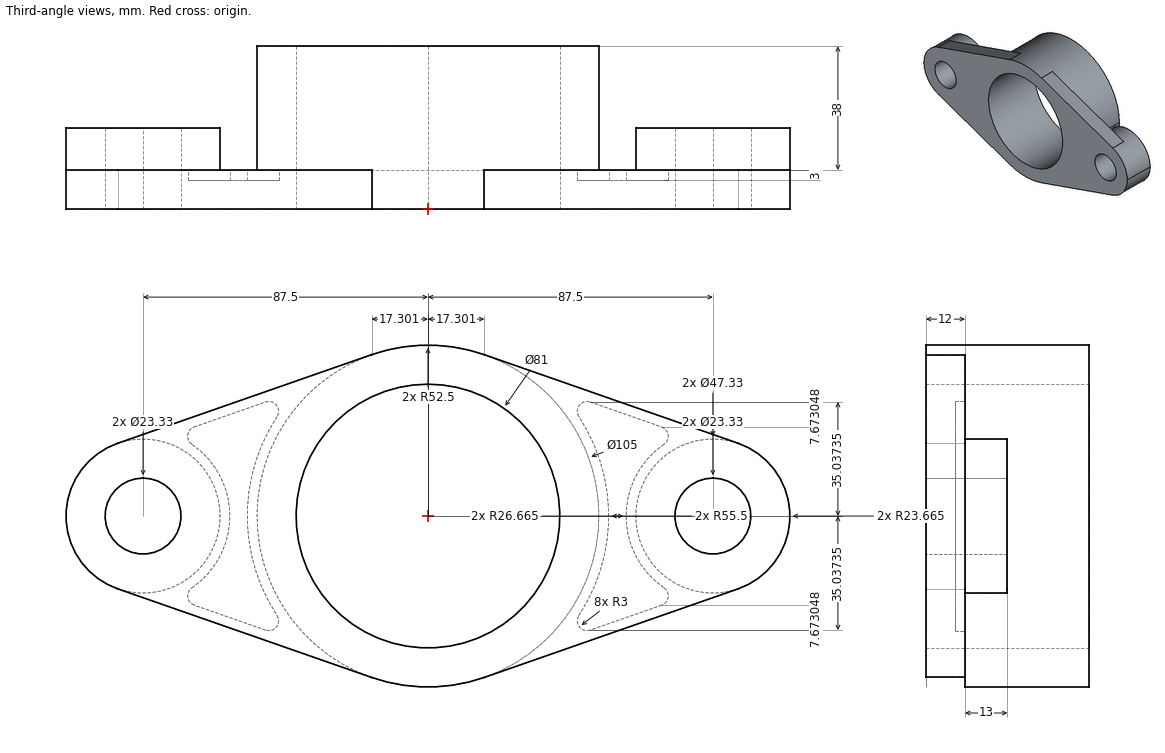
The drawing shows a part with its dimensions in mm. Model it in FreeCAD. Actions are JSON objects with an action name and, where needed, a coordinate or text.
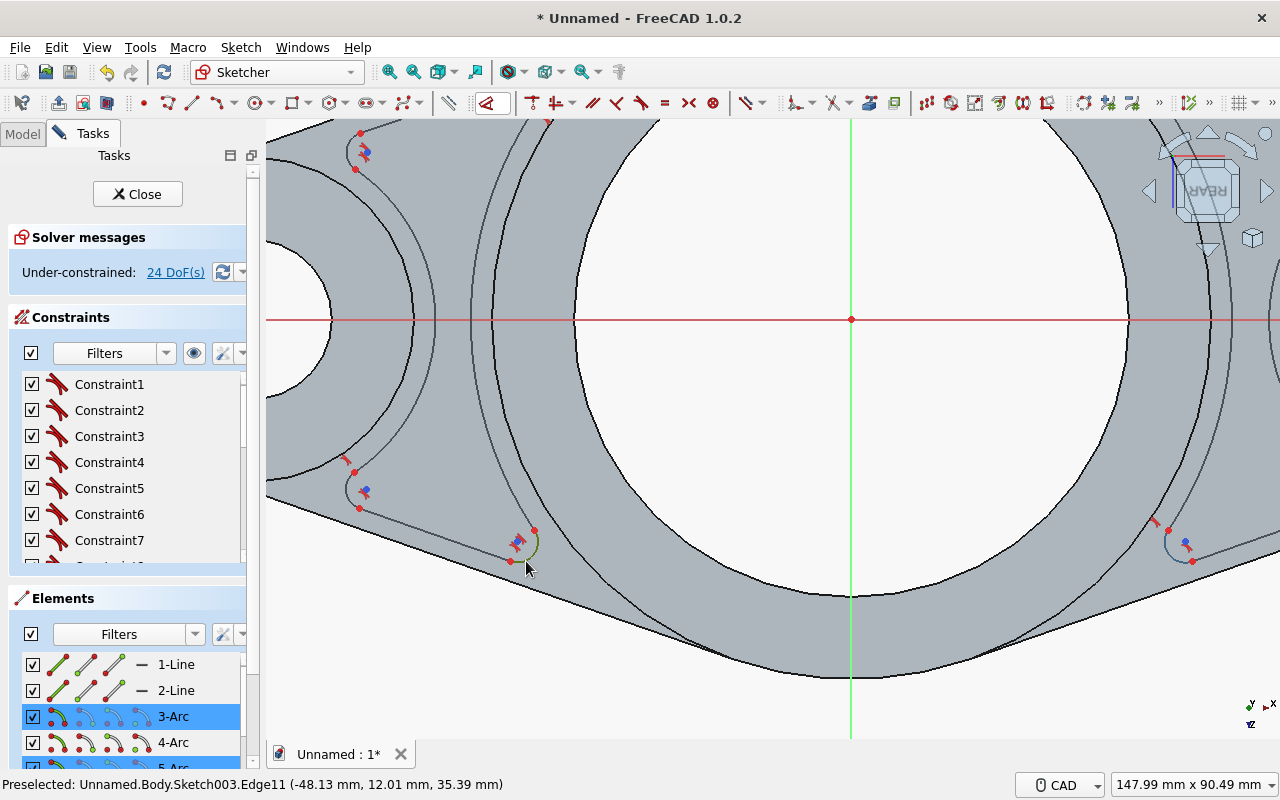
{"action": "scroll", "coordinate": [526, 562], "scroll_direction": "down", "scroll_amount": 3}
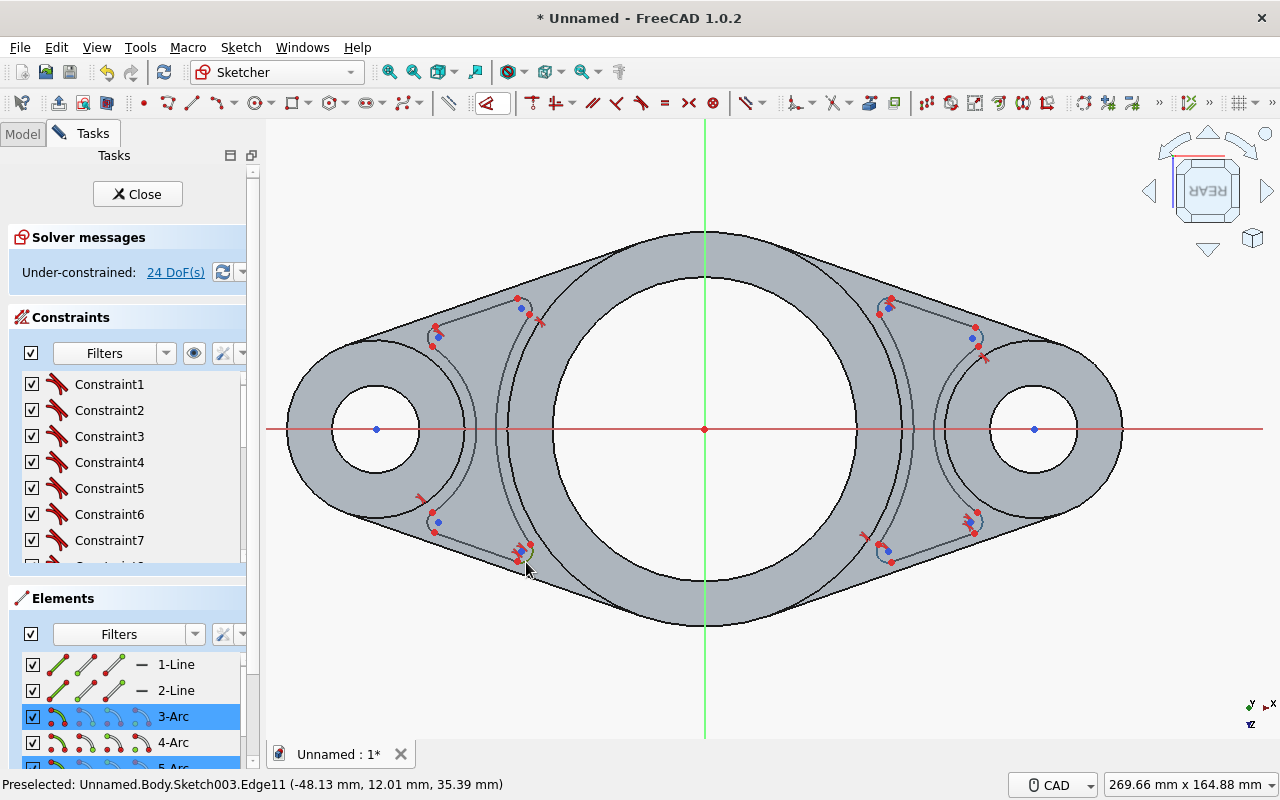
{"action": "scroll", "coordinate": [532, 307], "scroll_direction": "up", "scroll_amount": 3}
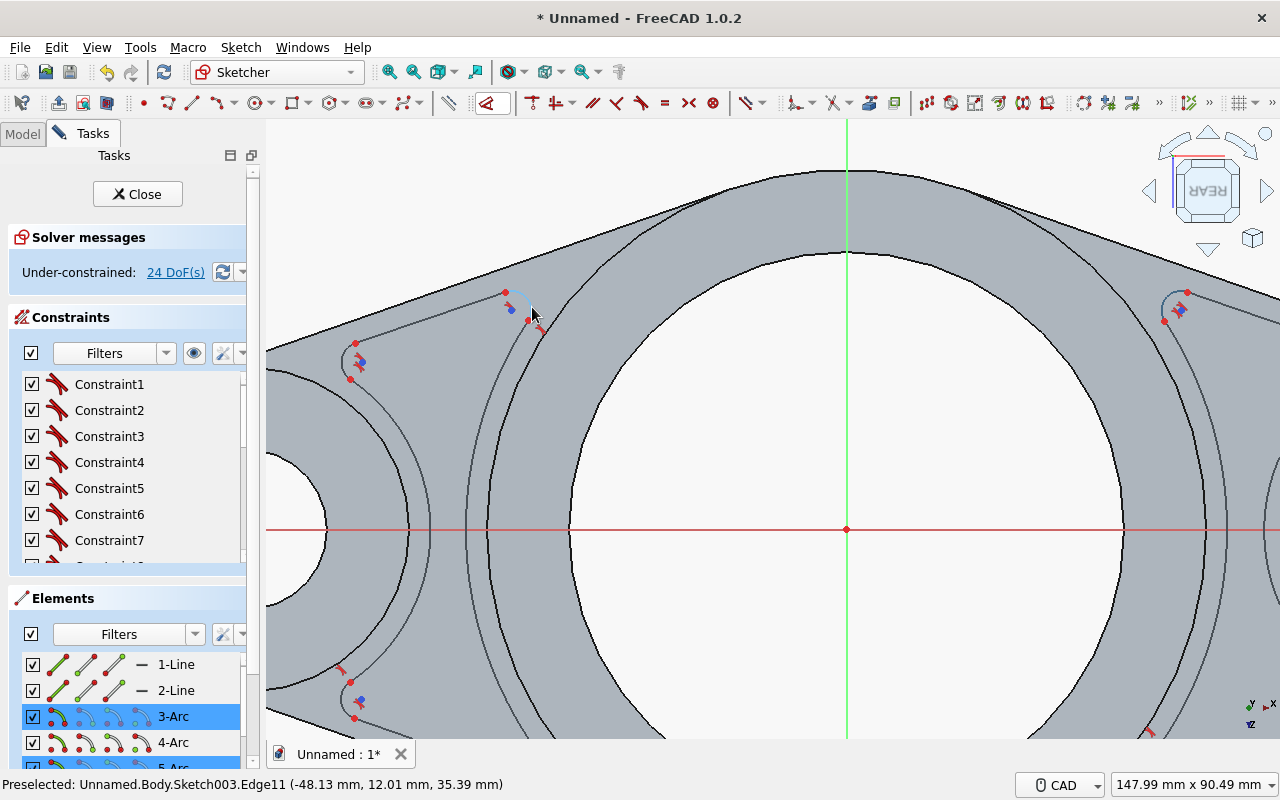
{"action": "left_click", "coordinate": [531, 307]}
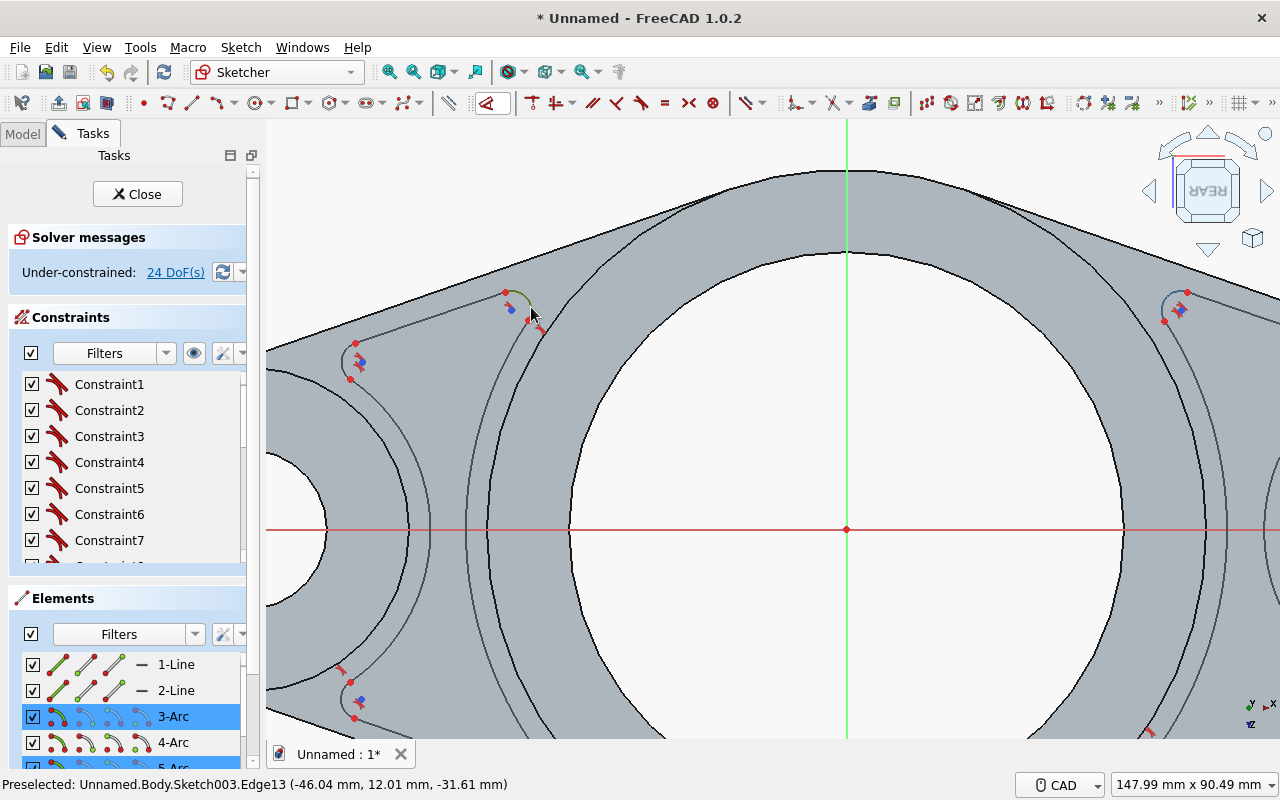
{"action": "left_click", "coordinate": [345, 351]}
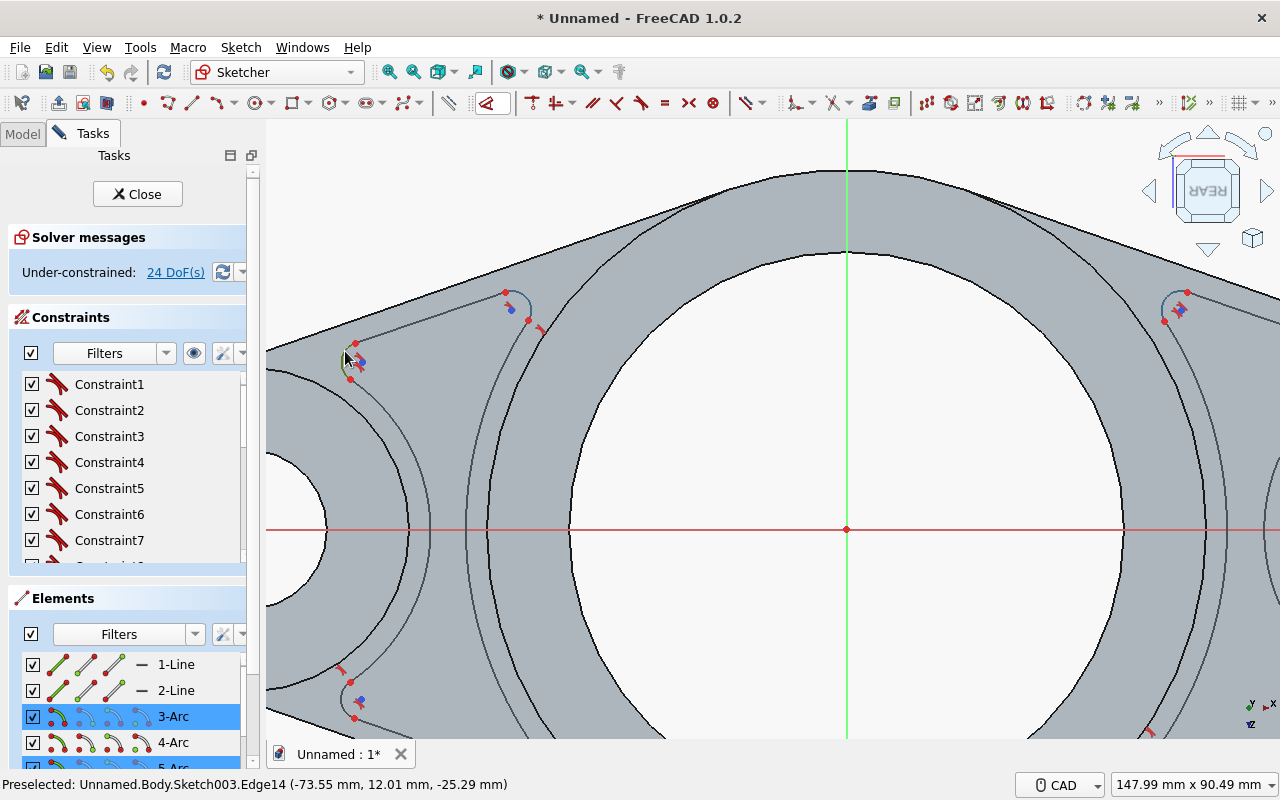
{"action": "left_click", "coordinate": [342, 693]}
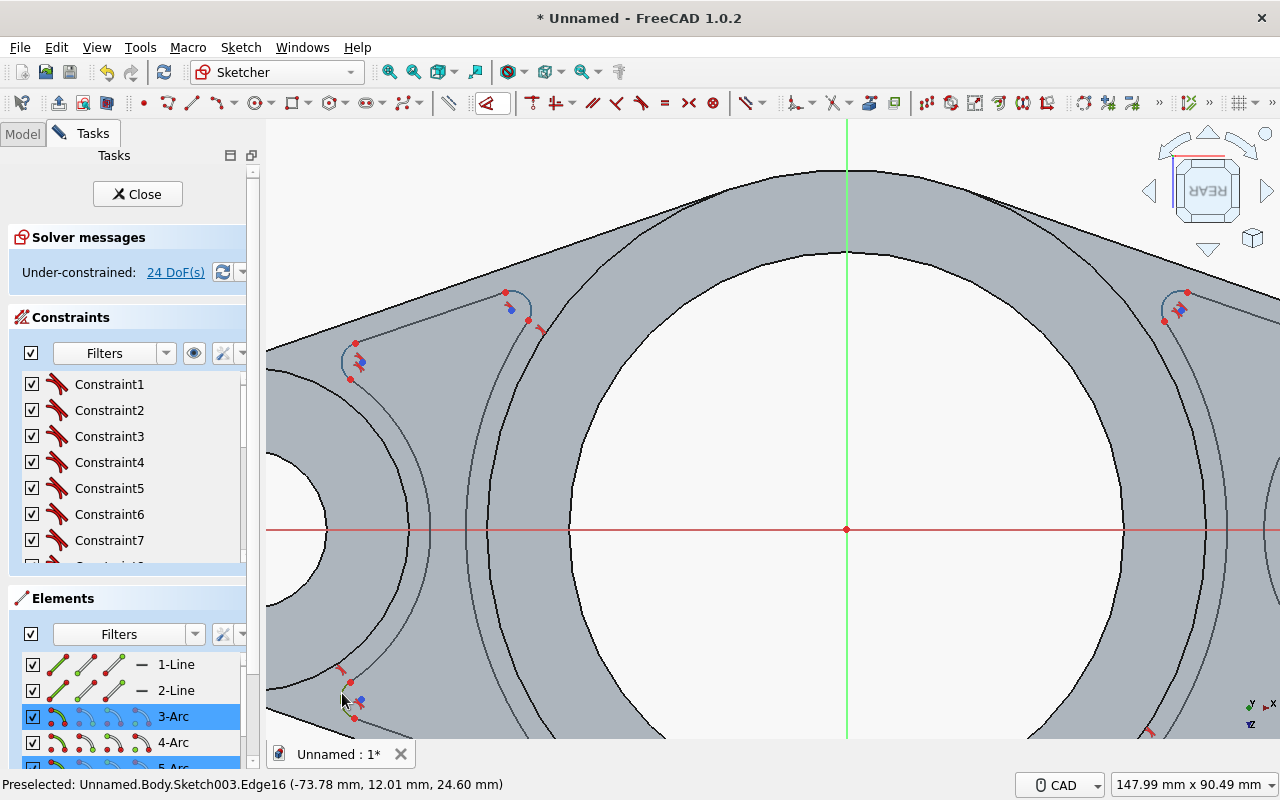
{"action": "left_click", "coordinate": [666, 104]}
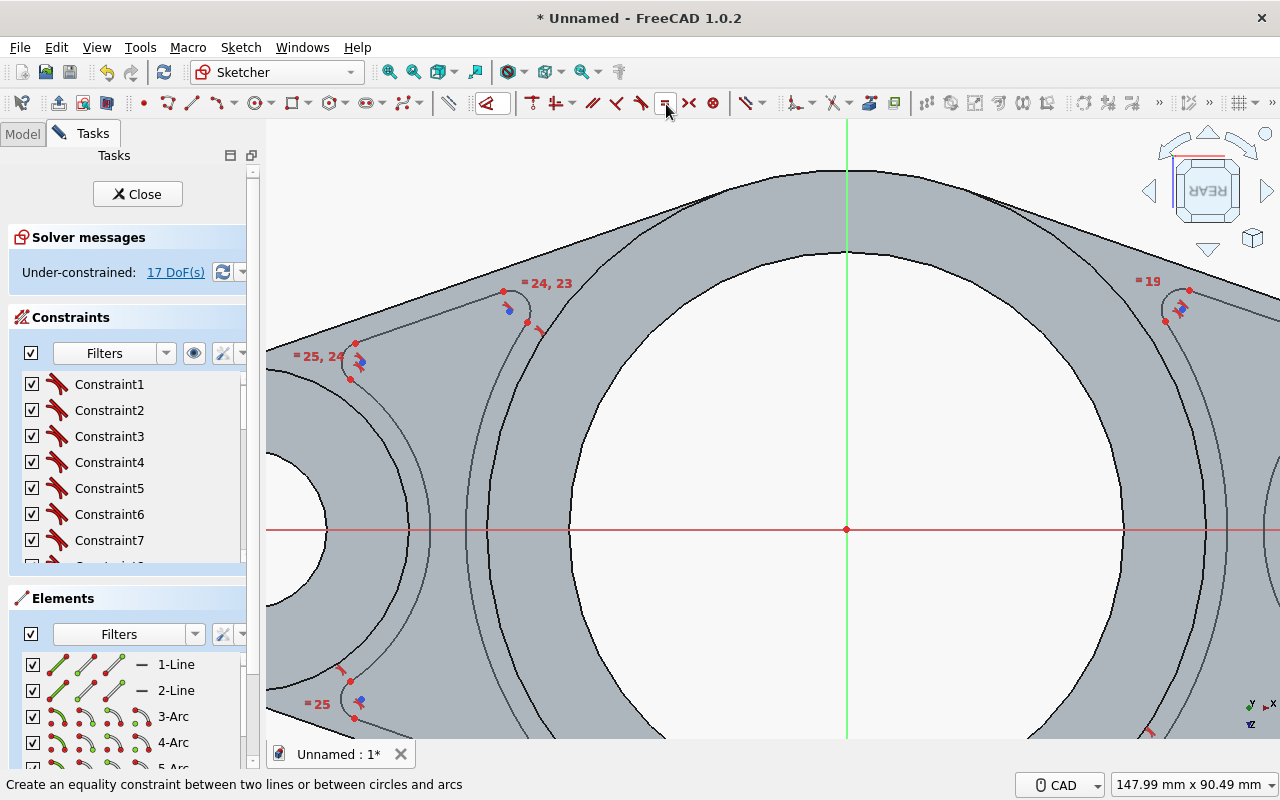
{"action": "scroll", "coordinate": [532, 307], "scroll_direction": "down", "scroll_amount": 3}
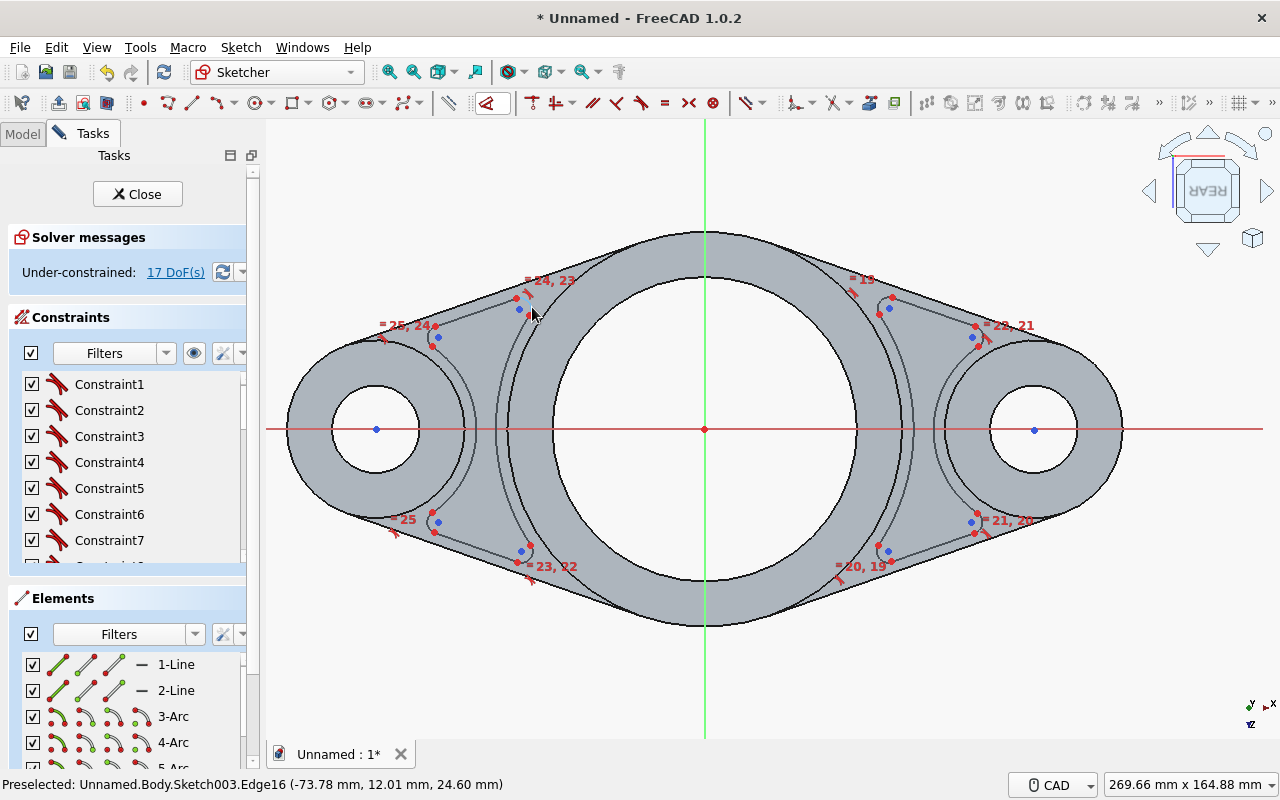
{"action": "left_click", "coordinate": [908, 478]}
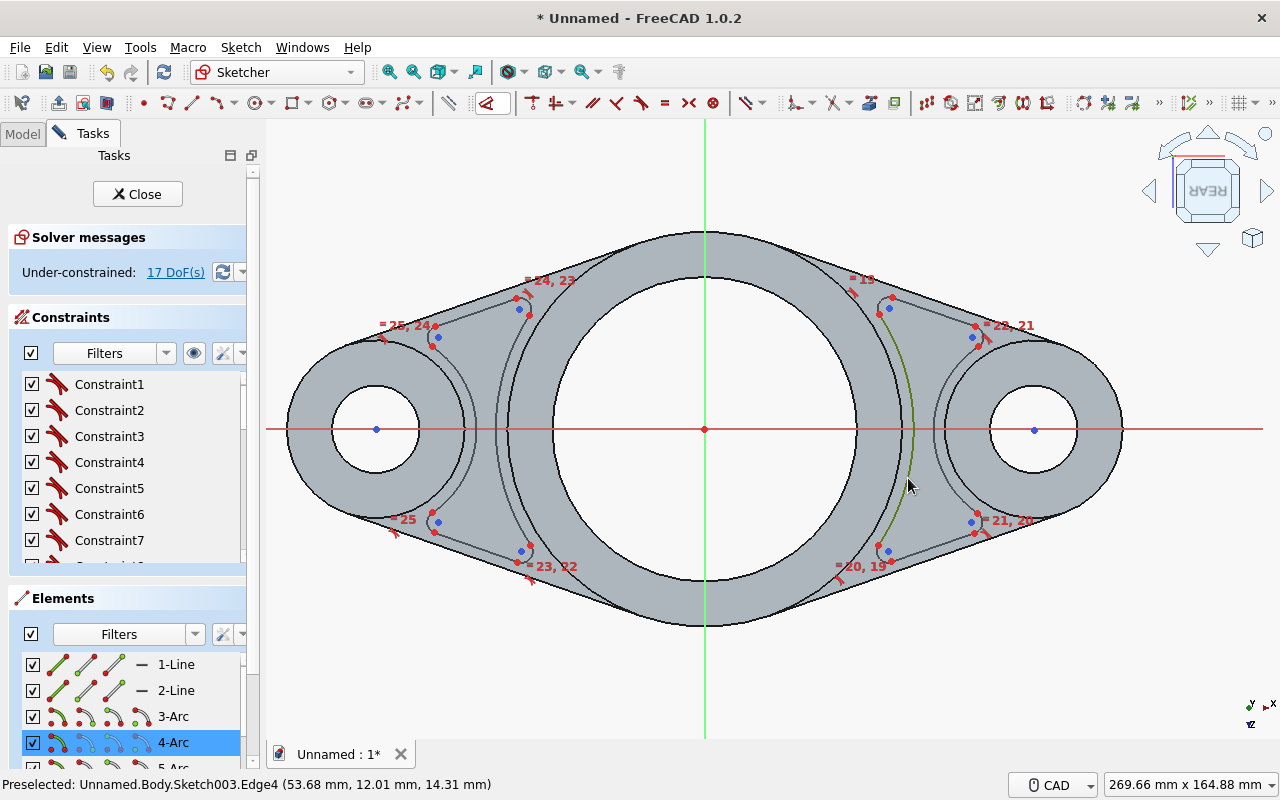
{"action": "left_click", "coordinate": [501, 382]}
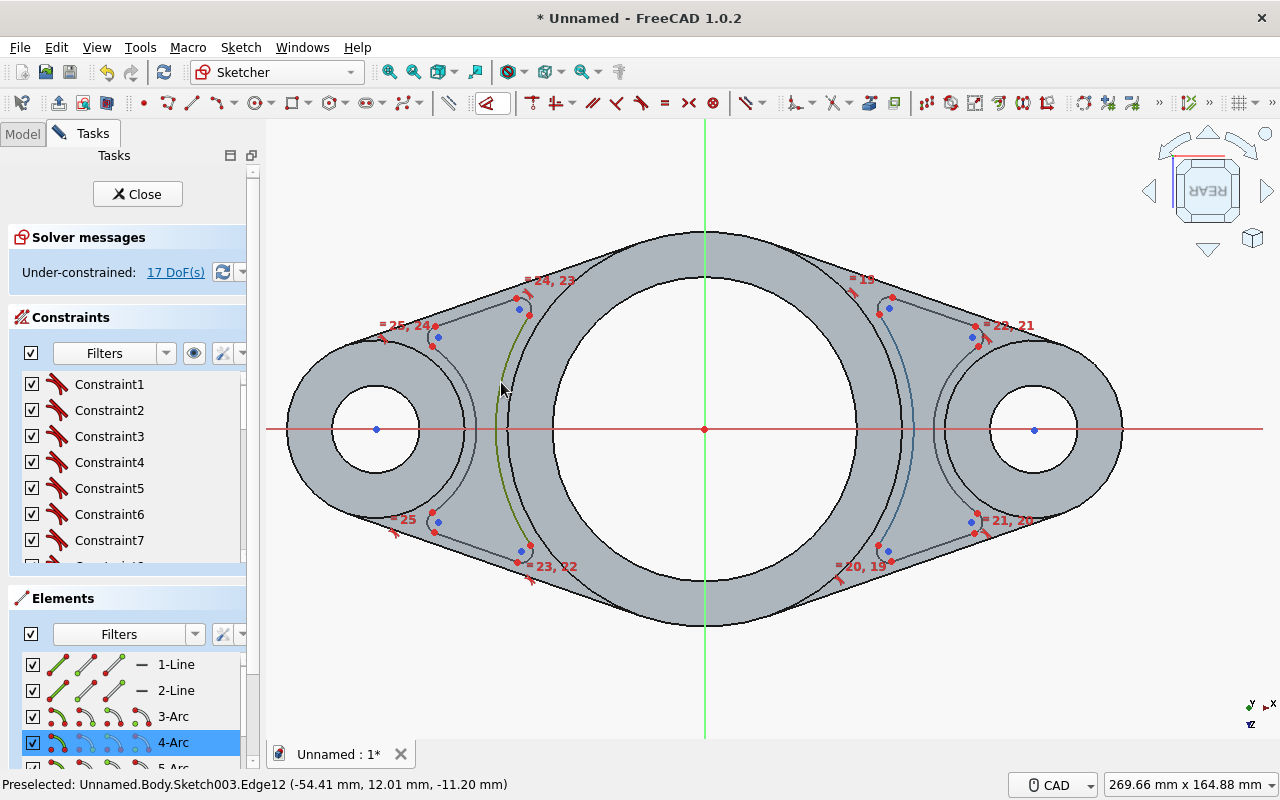
{"action": "left_click", "coordinate": [666, 104]}